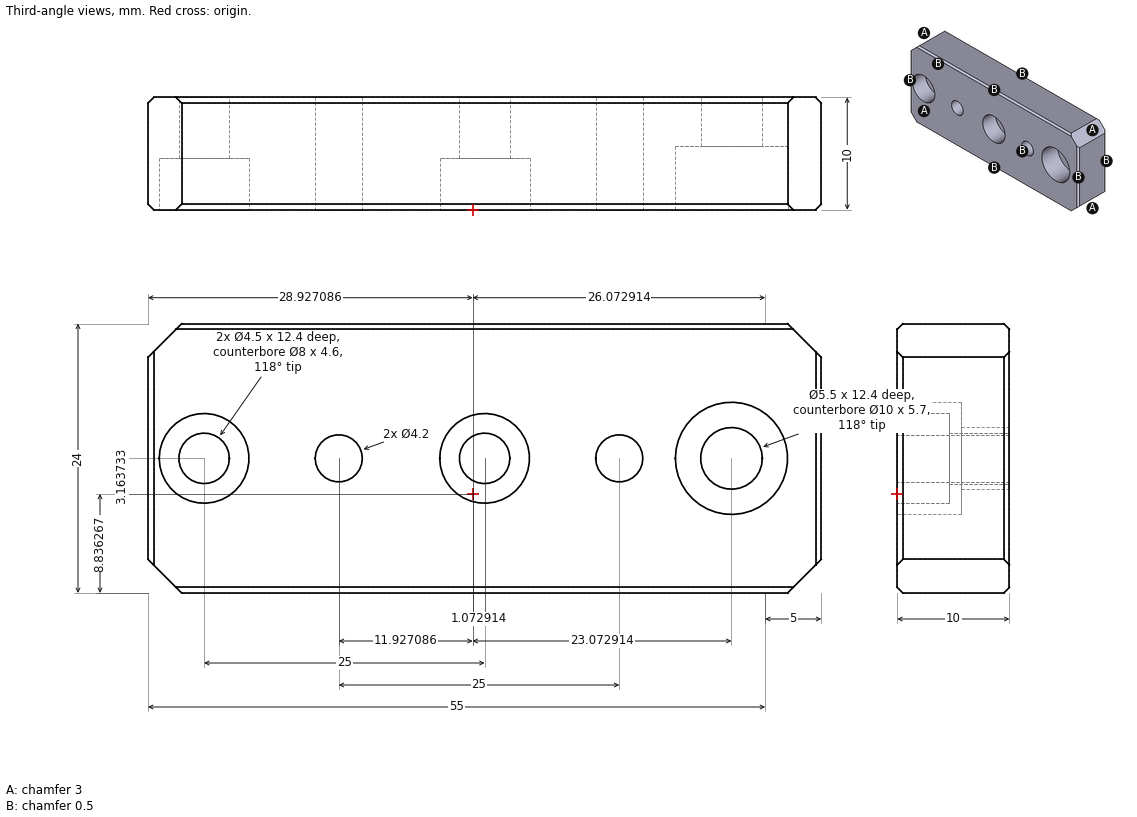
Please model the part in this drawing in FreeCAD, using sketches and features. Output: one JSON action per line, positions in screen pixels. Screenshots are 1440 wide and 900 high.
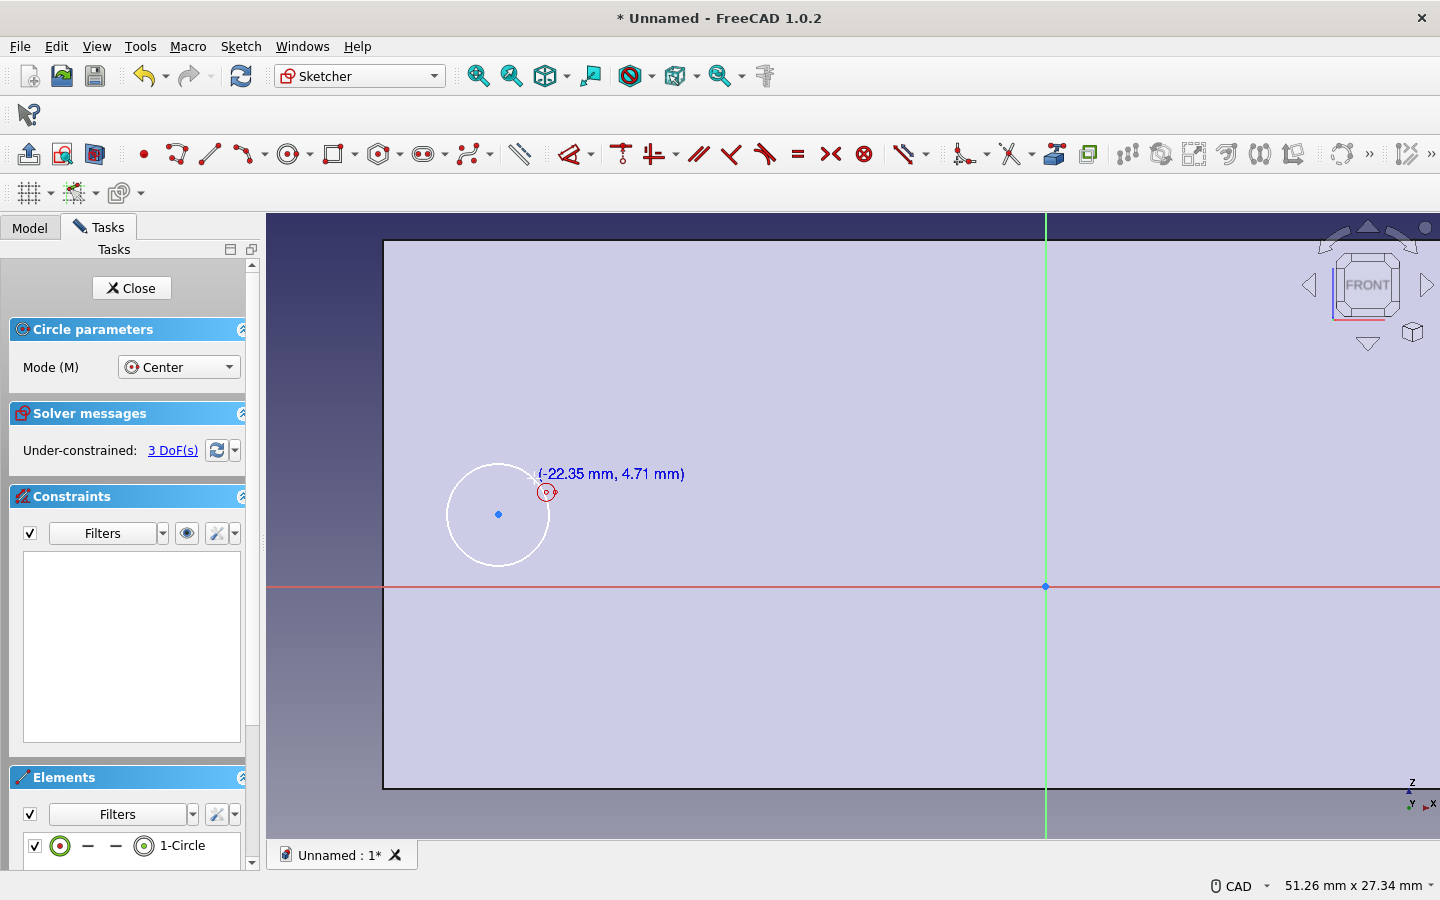
{"action": "left_click", "coordinate": [1070, 514]}
{"action": "left_click", "coordinate": [1107, 478]}
{"action": "key", "text": "Escape"}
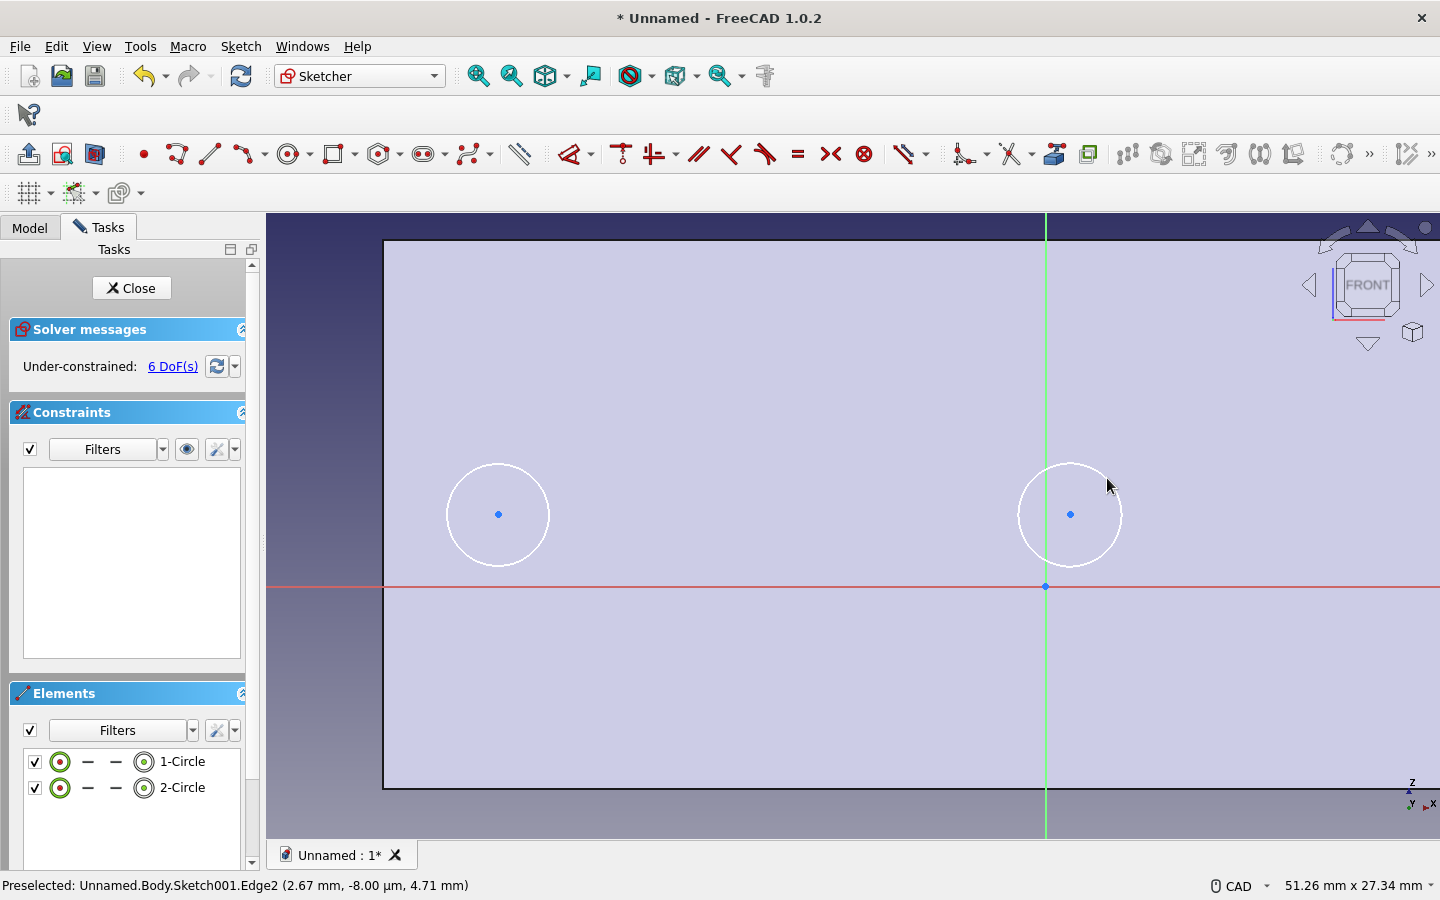
{"action": "left_click", "coordinate": [534, 479]}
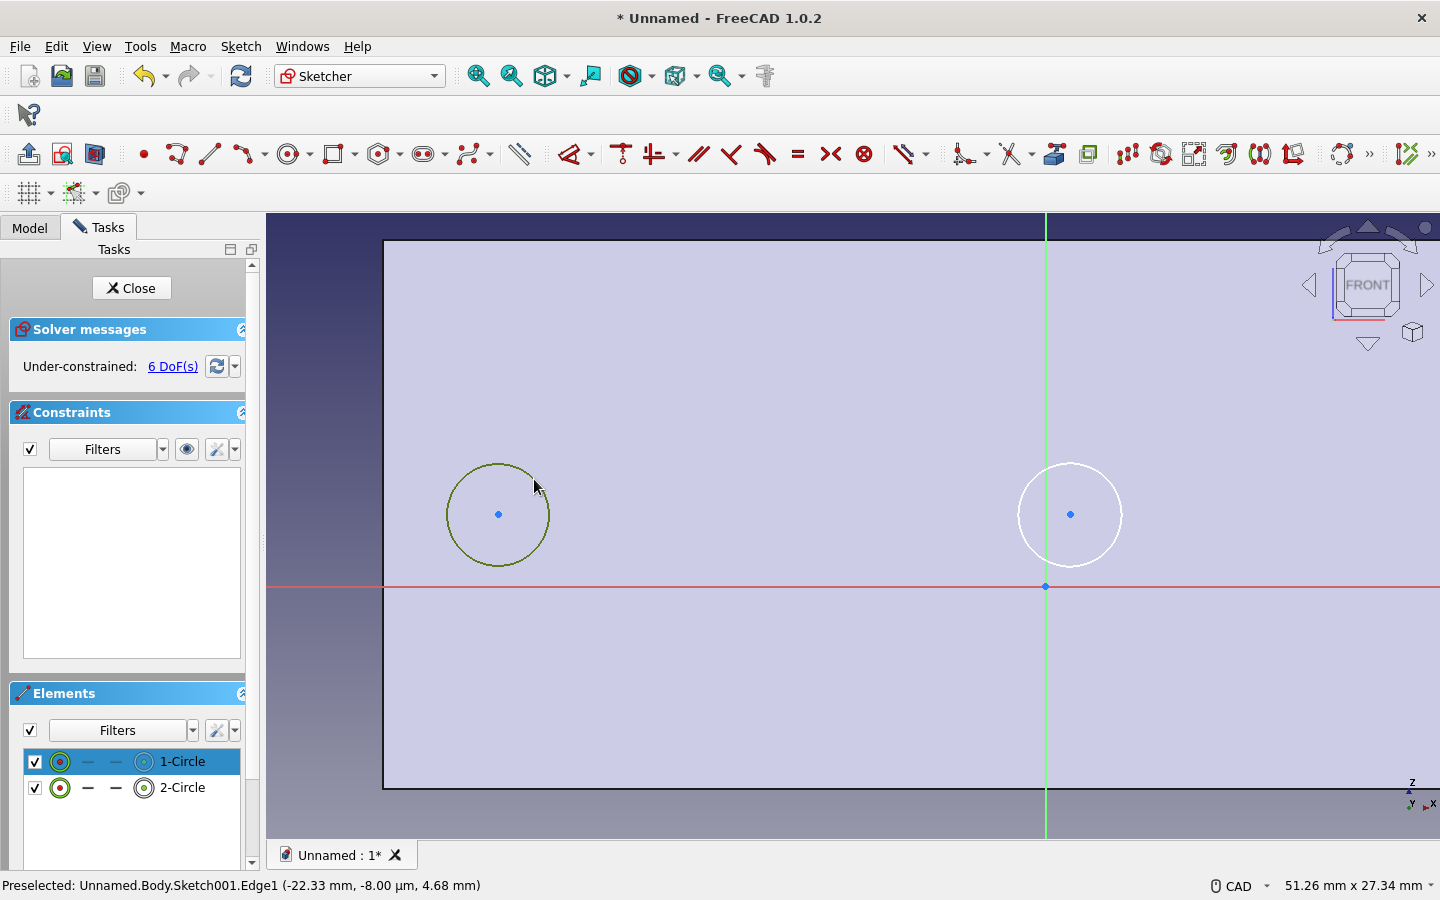
{"action": "left_click", "coordinate": [1106, 478]}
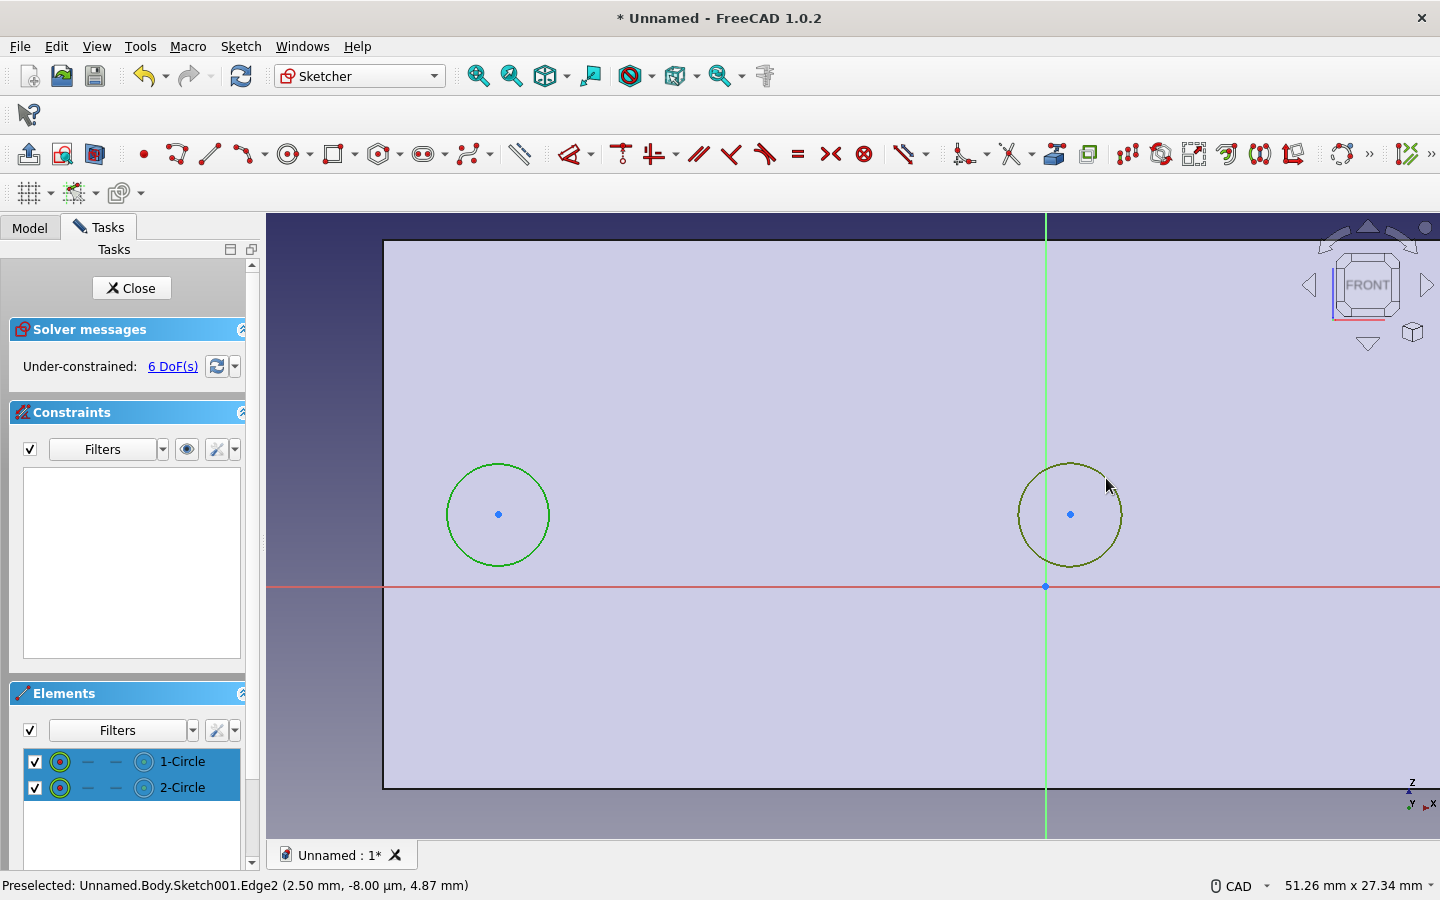
{"action": "key", "text": "e"}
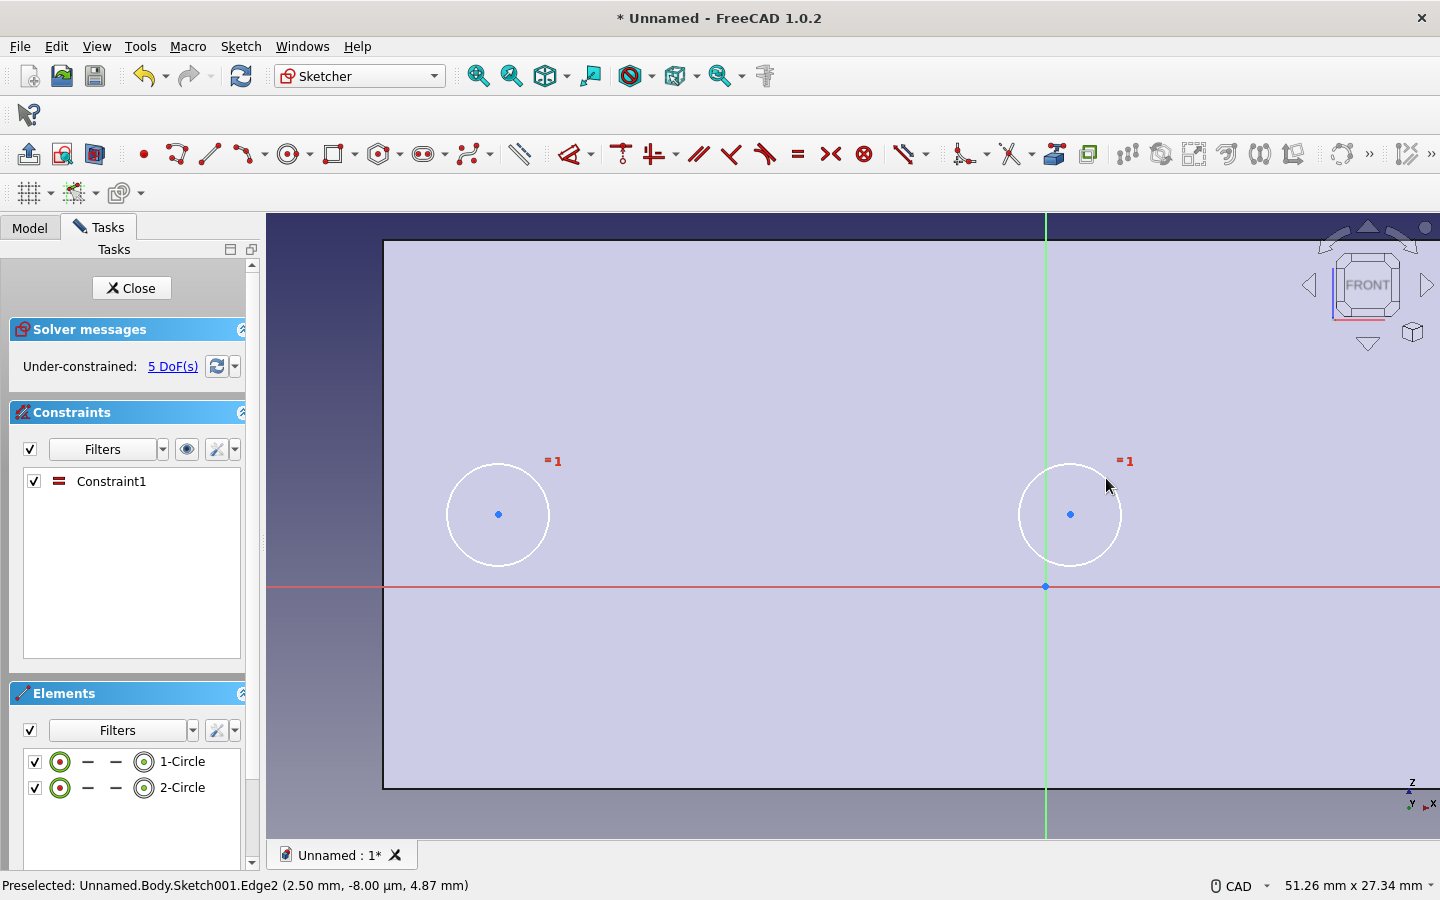
{"action": "left_click", "coordinate": [498, 515]}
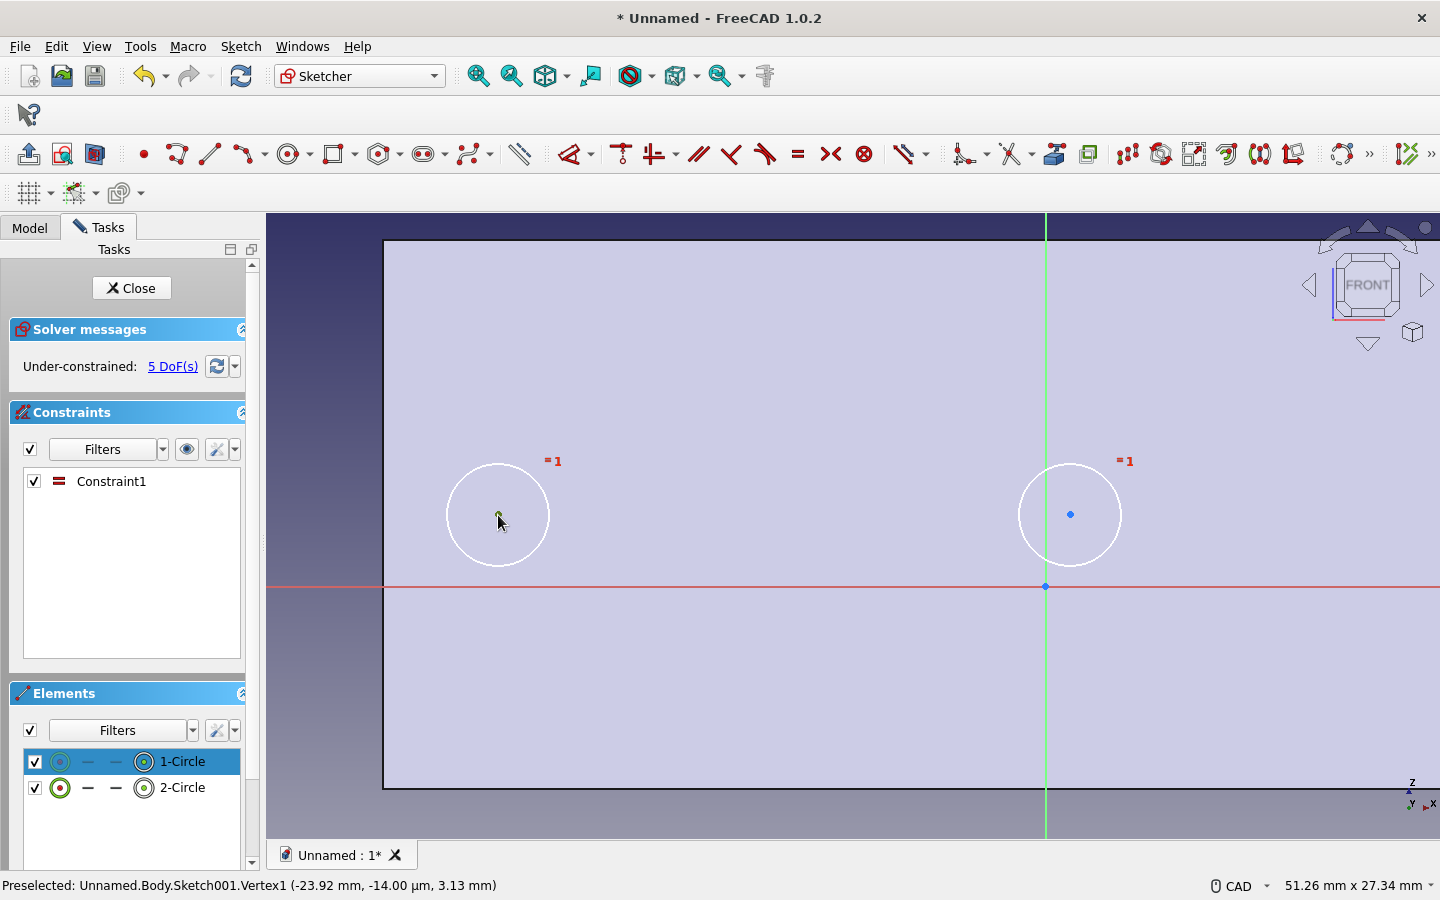
{"action": "left_click", "coordinate": [1070, 515]}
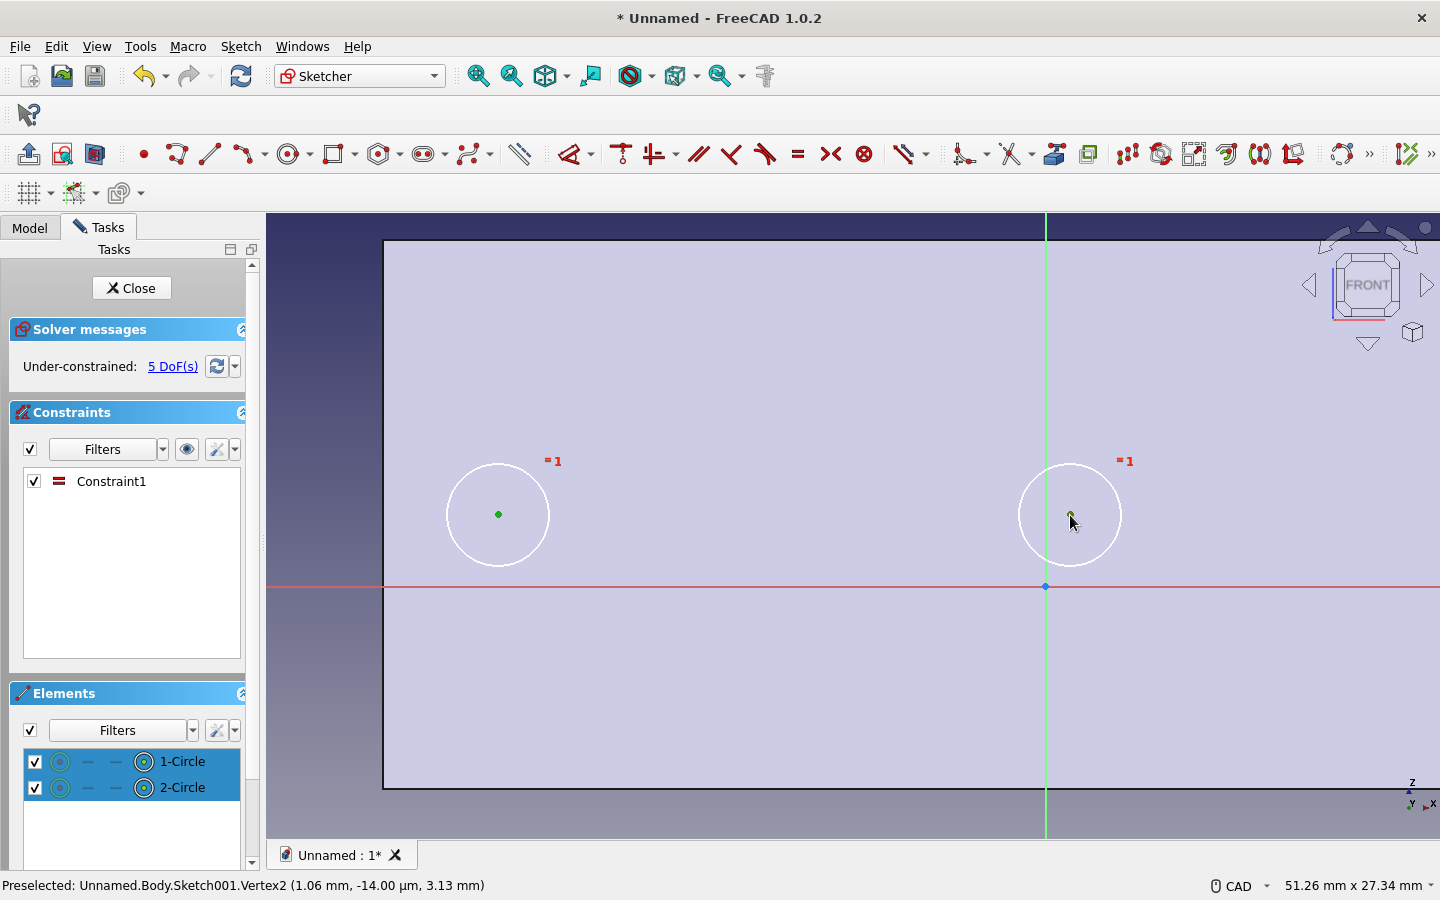
{"action": "key", "text": "h"}